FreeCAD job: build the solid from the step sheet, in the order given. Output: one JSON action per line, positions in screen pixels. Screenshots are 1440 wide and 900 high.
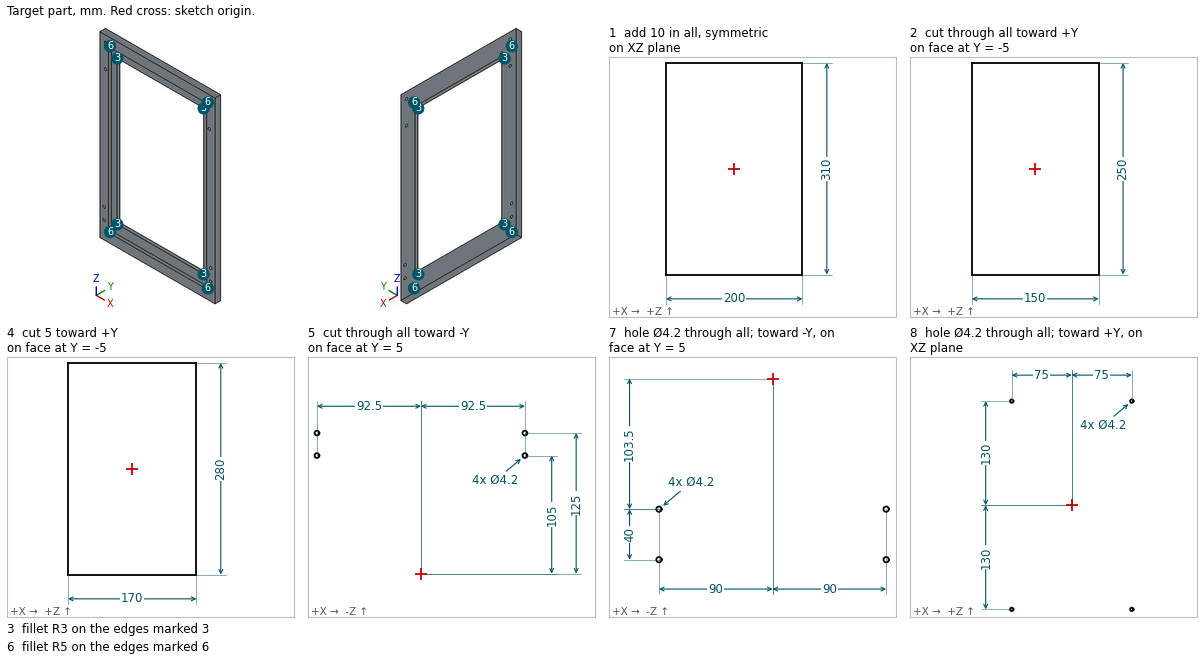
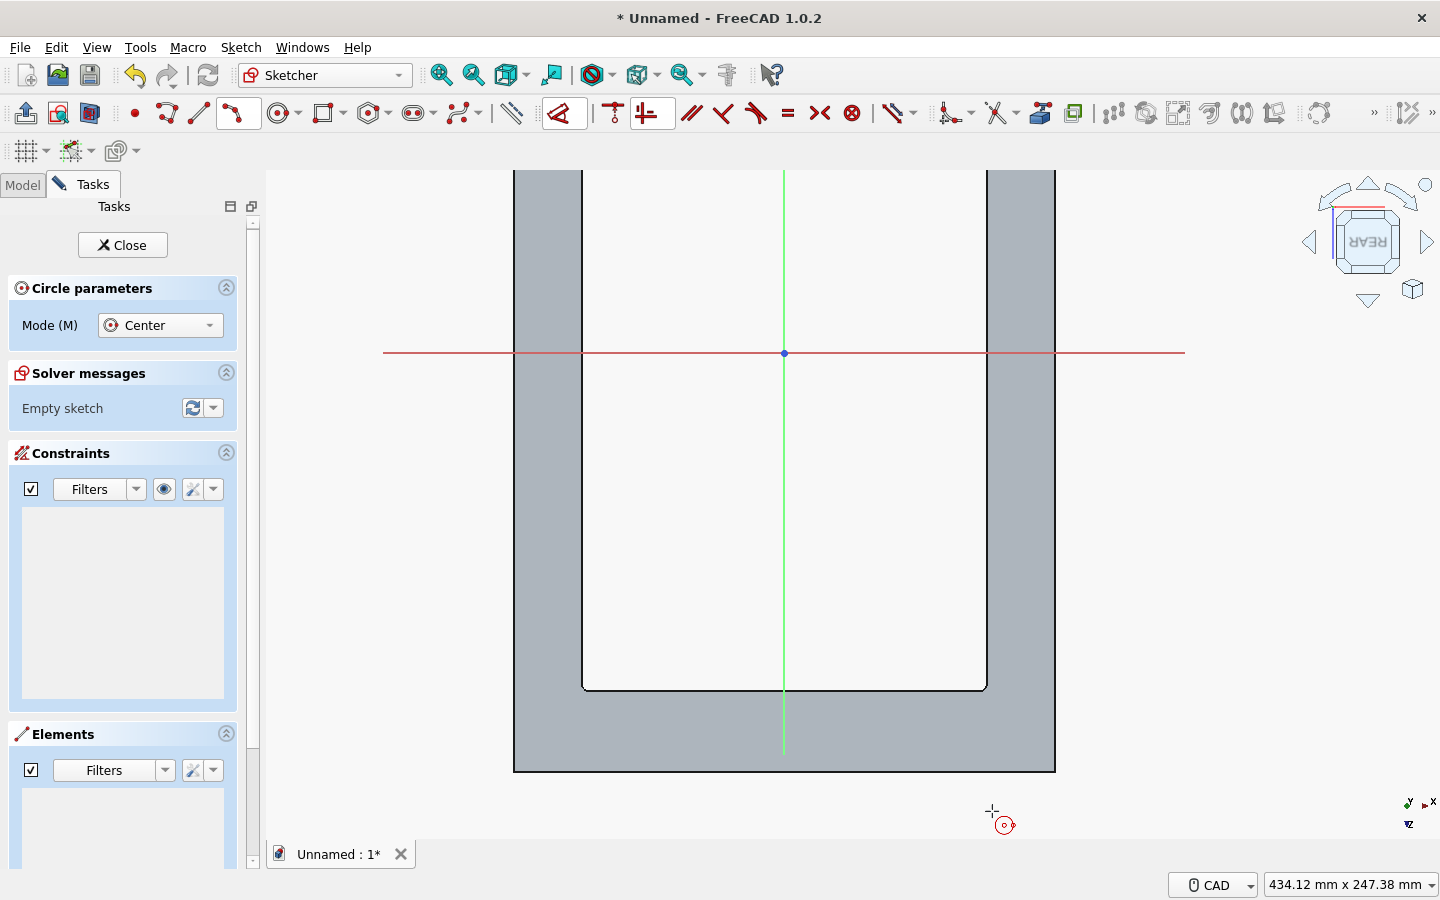
{"action": "scroll", "coordinate": [541, 633], "scroll_direction": "up", "scroll_amount": 7}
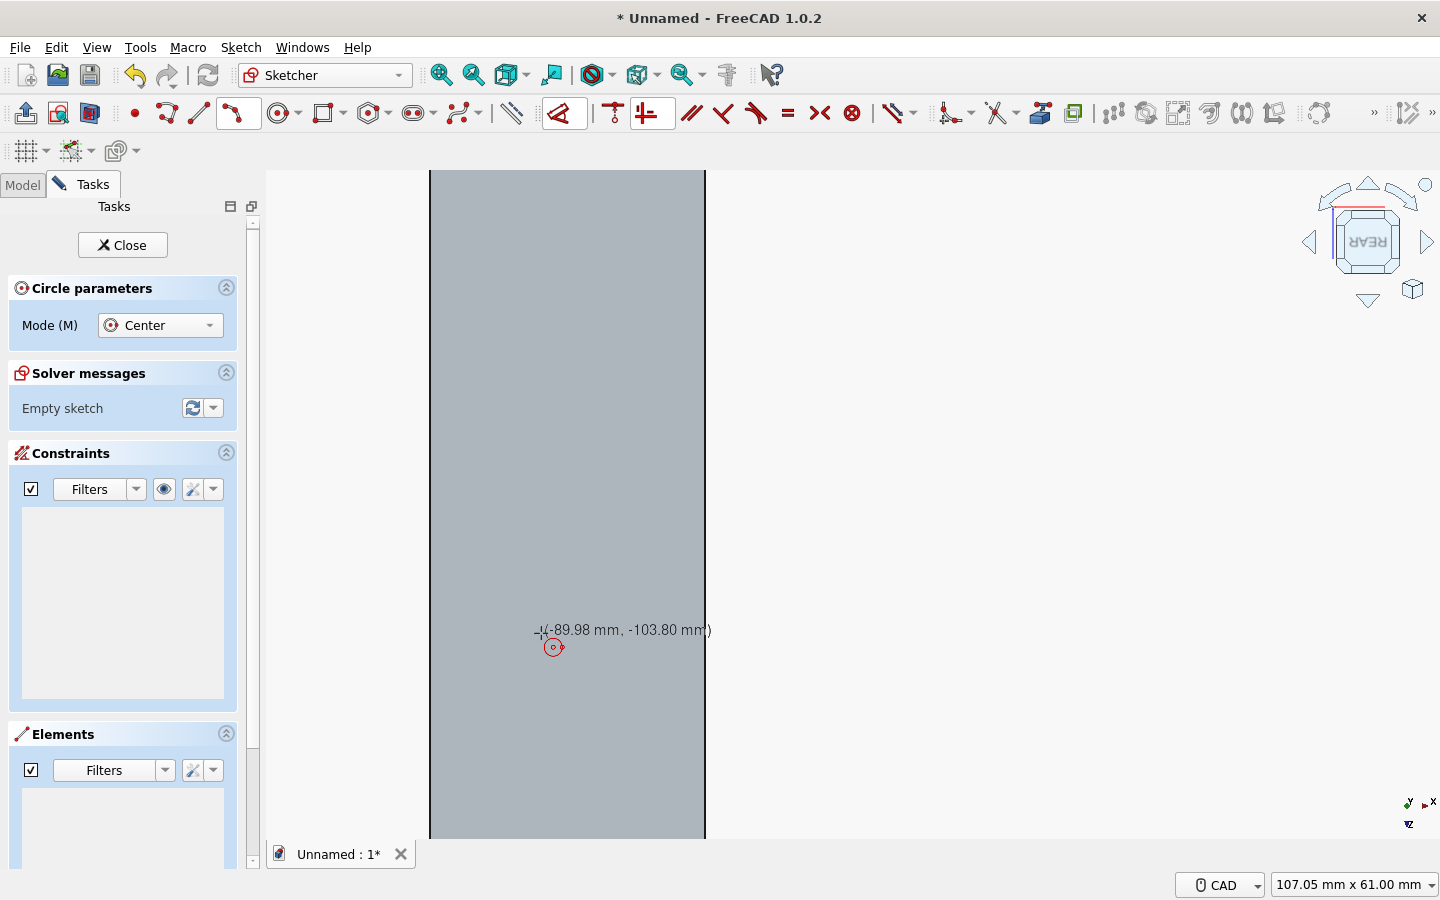
{"action": "scroll", "coordinate": [541, 573], "scroll_direction": "down", "scroll_amount": 7}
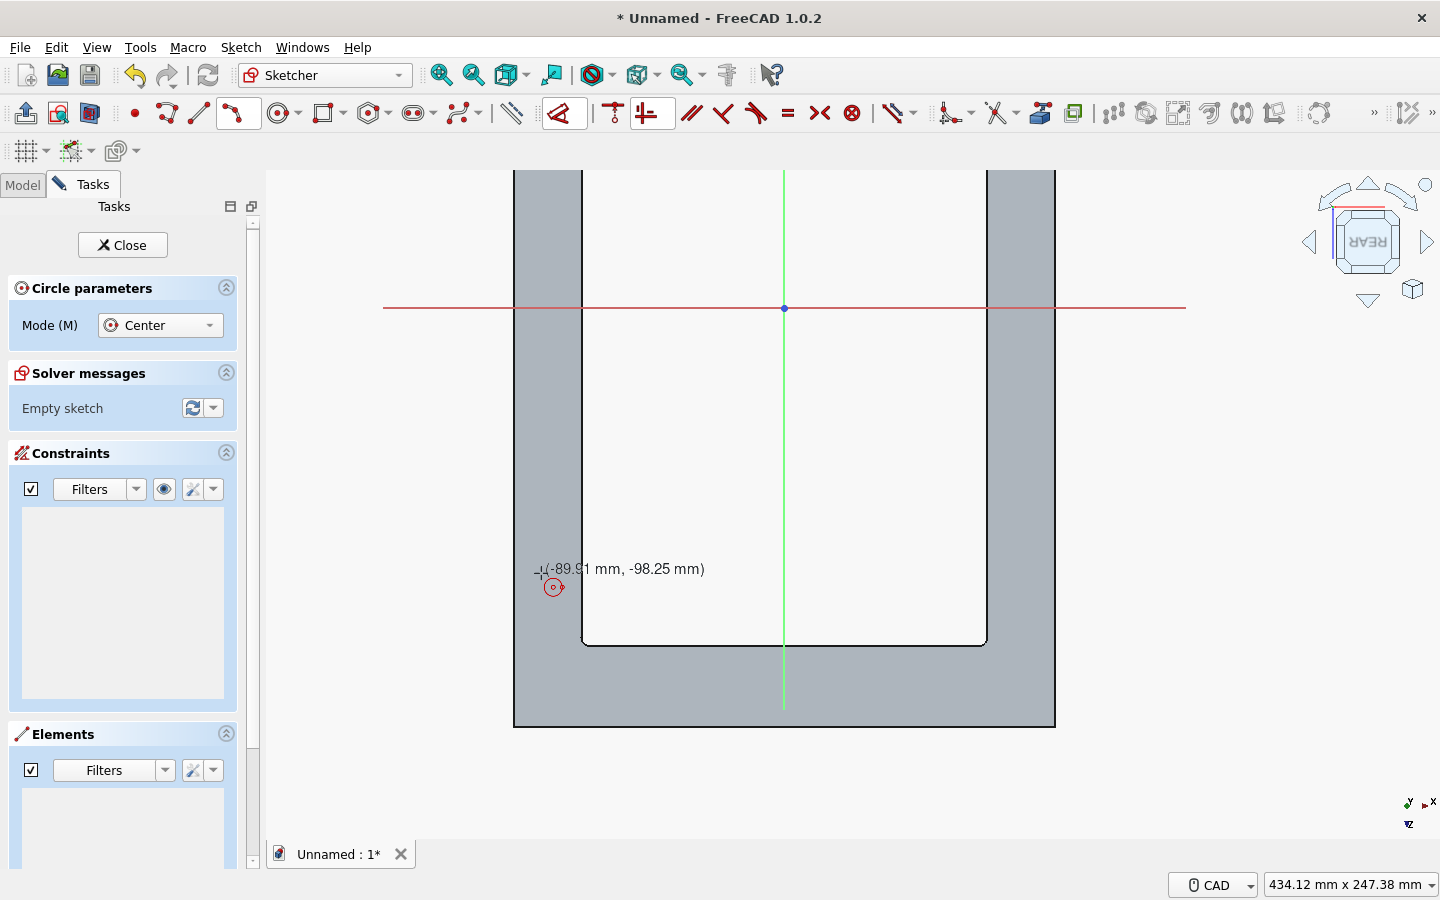
{"action": "left_click", "coordinate": [541, 588]}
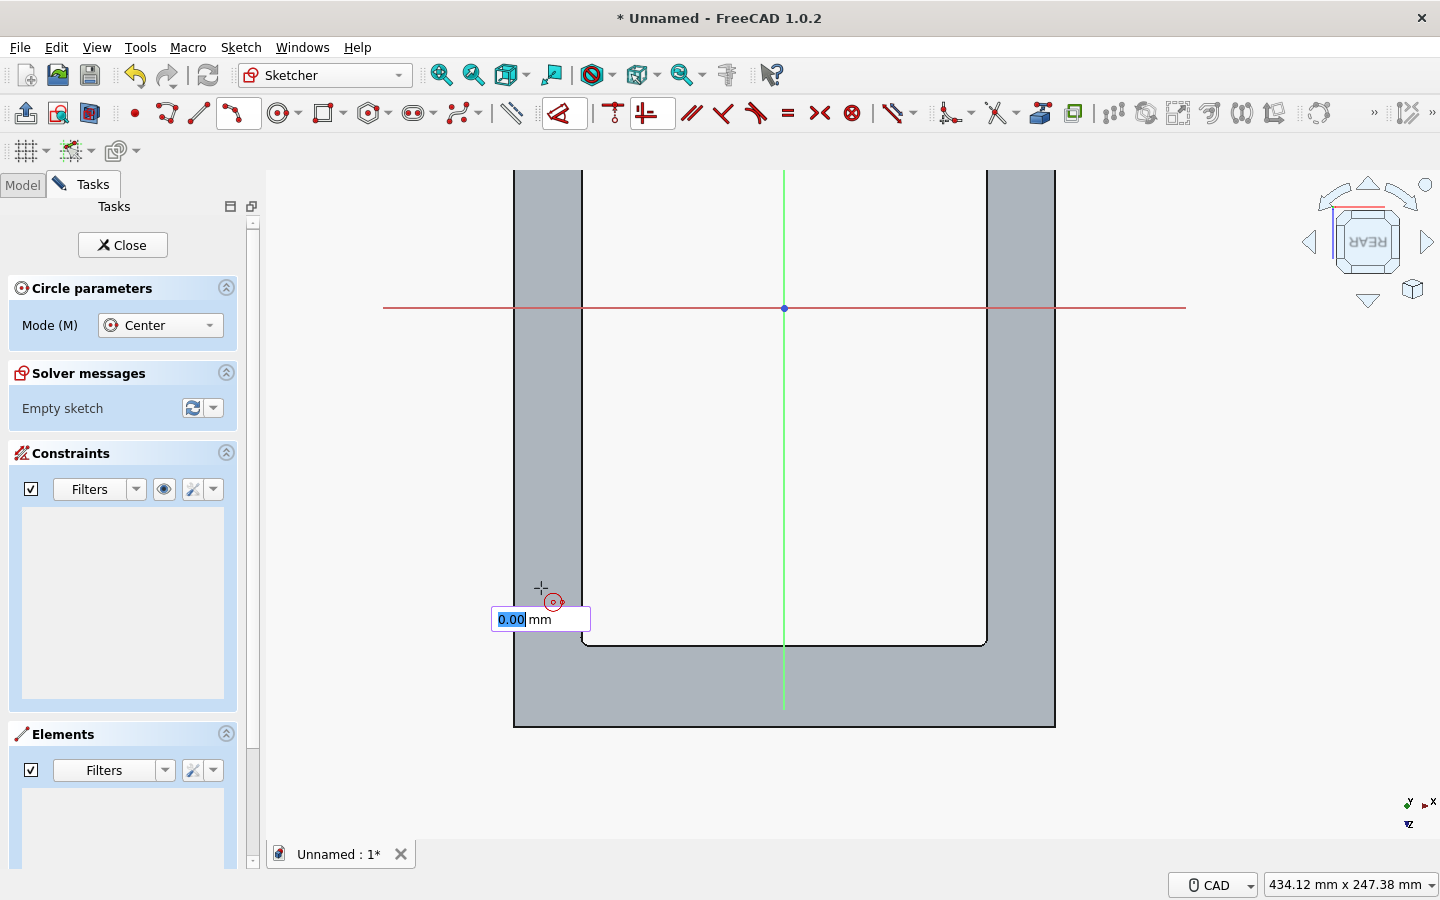
{"action": "scroll", "coordinate": [545, 584], "scroll_direction": "up", "scroll_amount": 6}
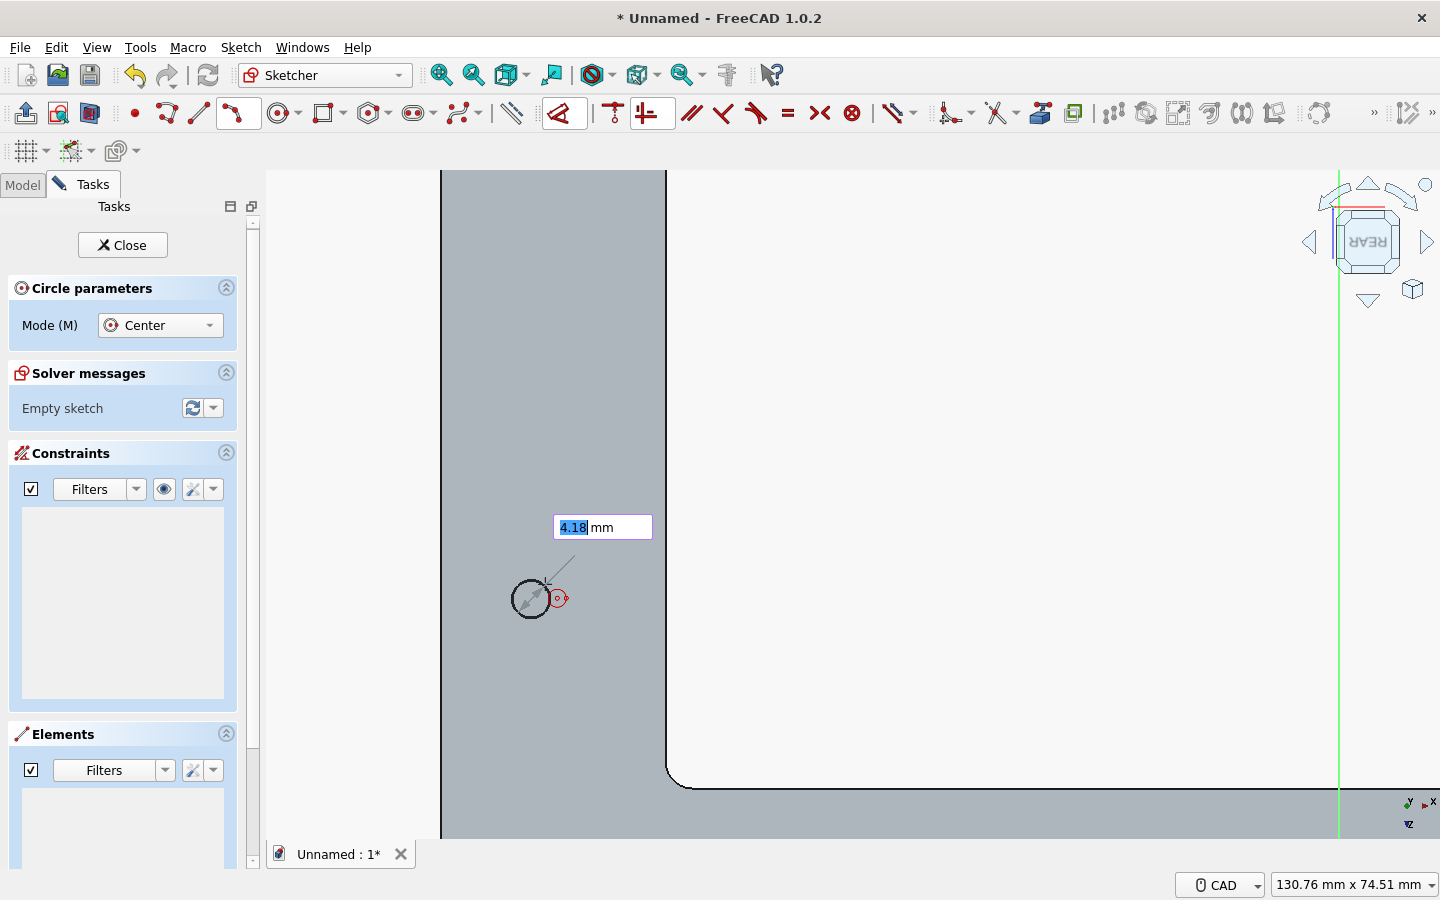
{"action": "left_click", "coordinate": [544, 582]}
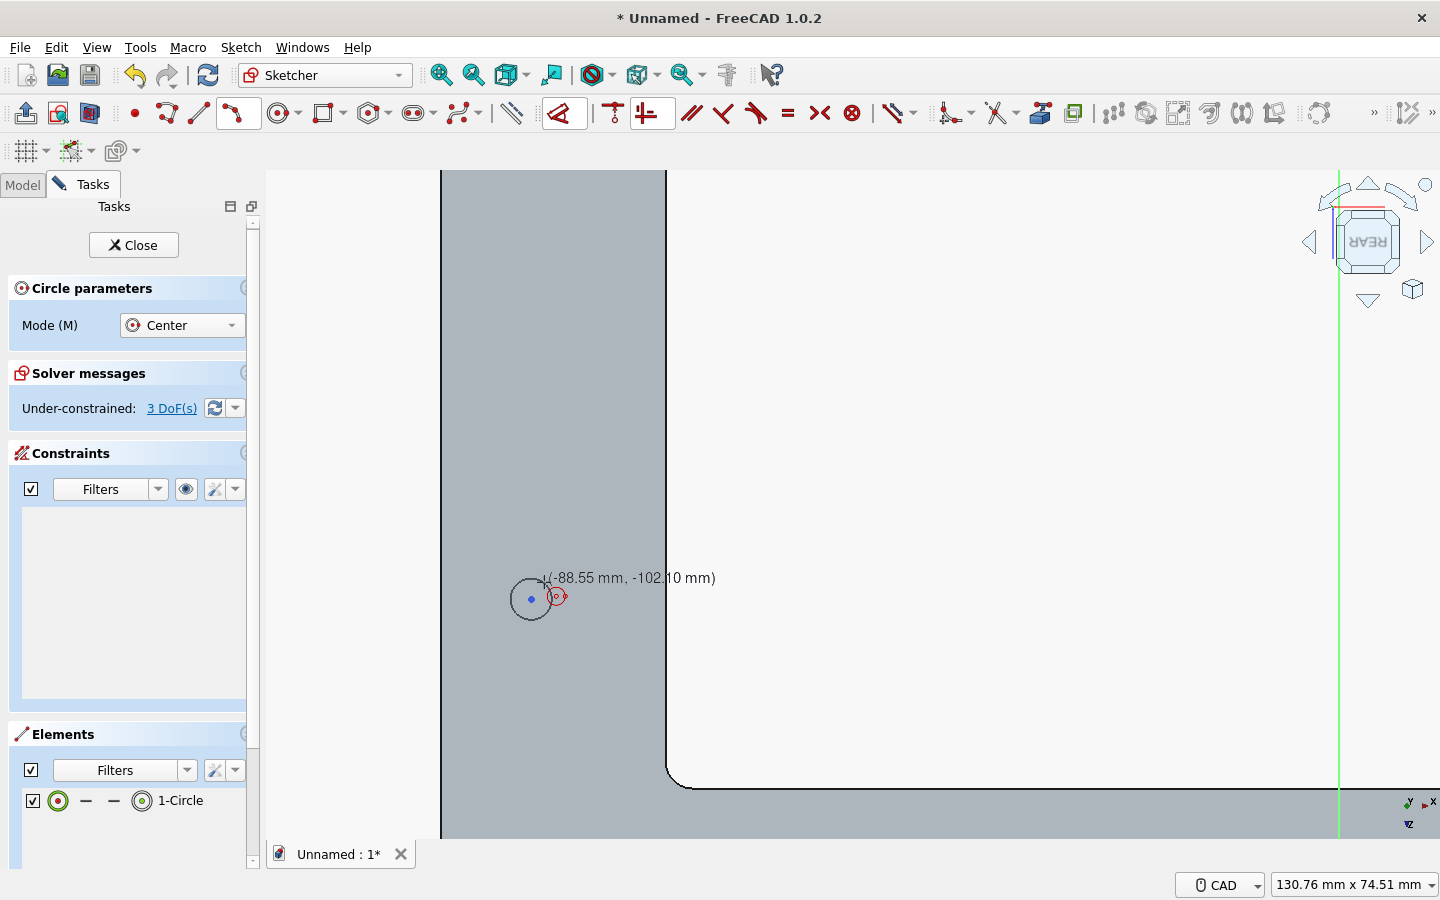
{"action": "scroll", "coordinate": [545, 584], "scroll_direction": "down", "scroll_amount": 6}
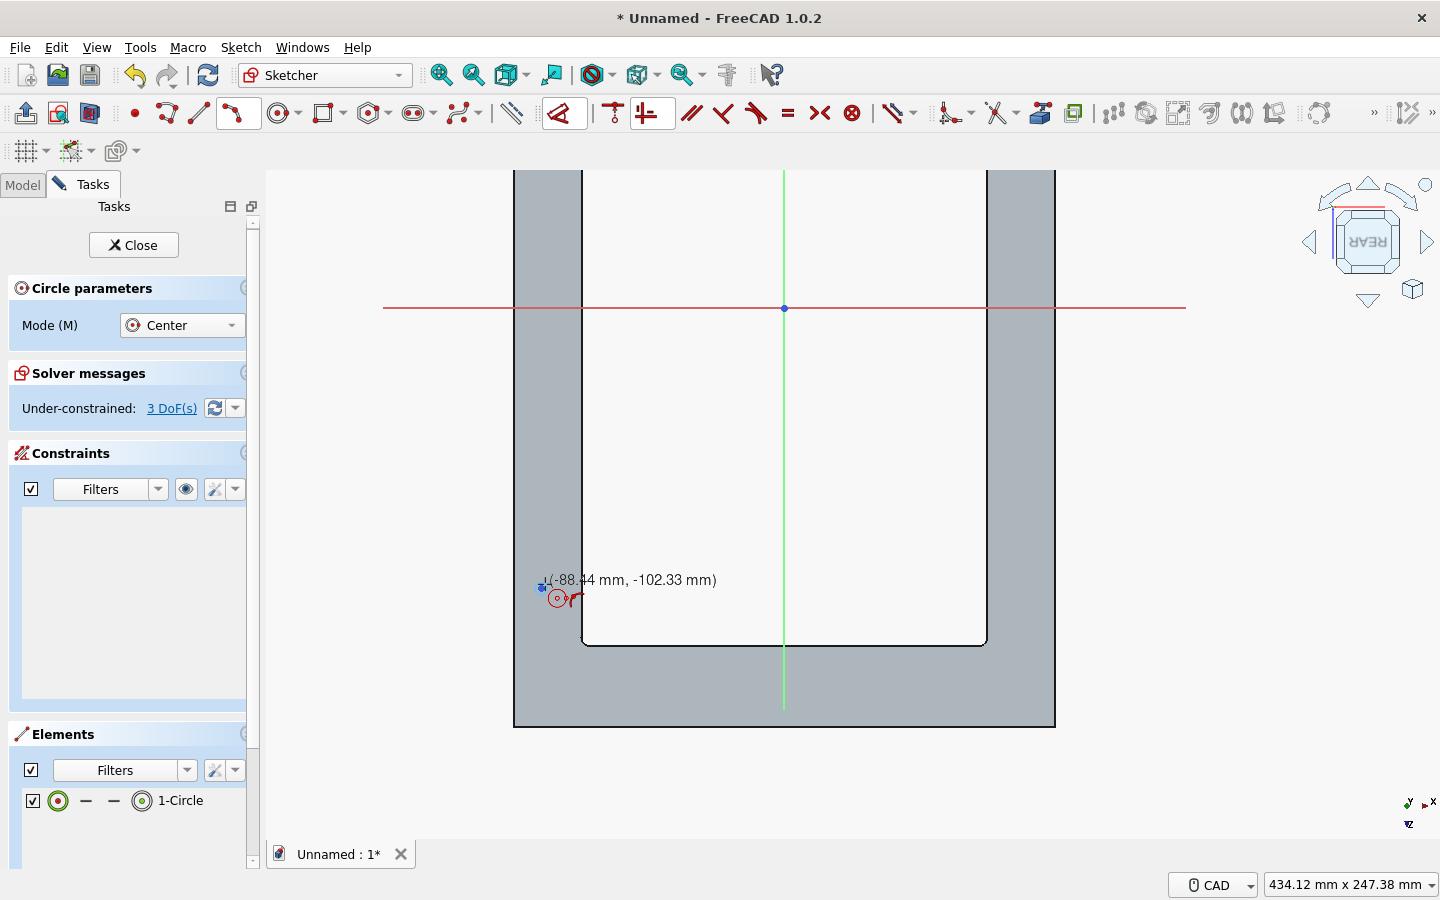
{"action": "scroll", "coordinate": [541, 696], "scroll_direction": "up", "scroll_amount": 7}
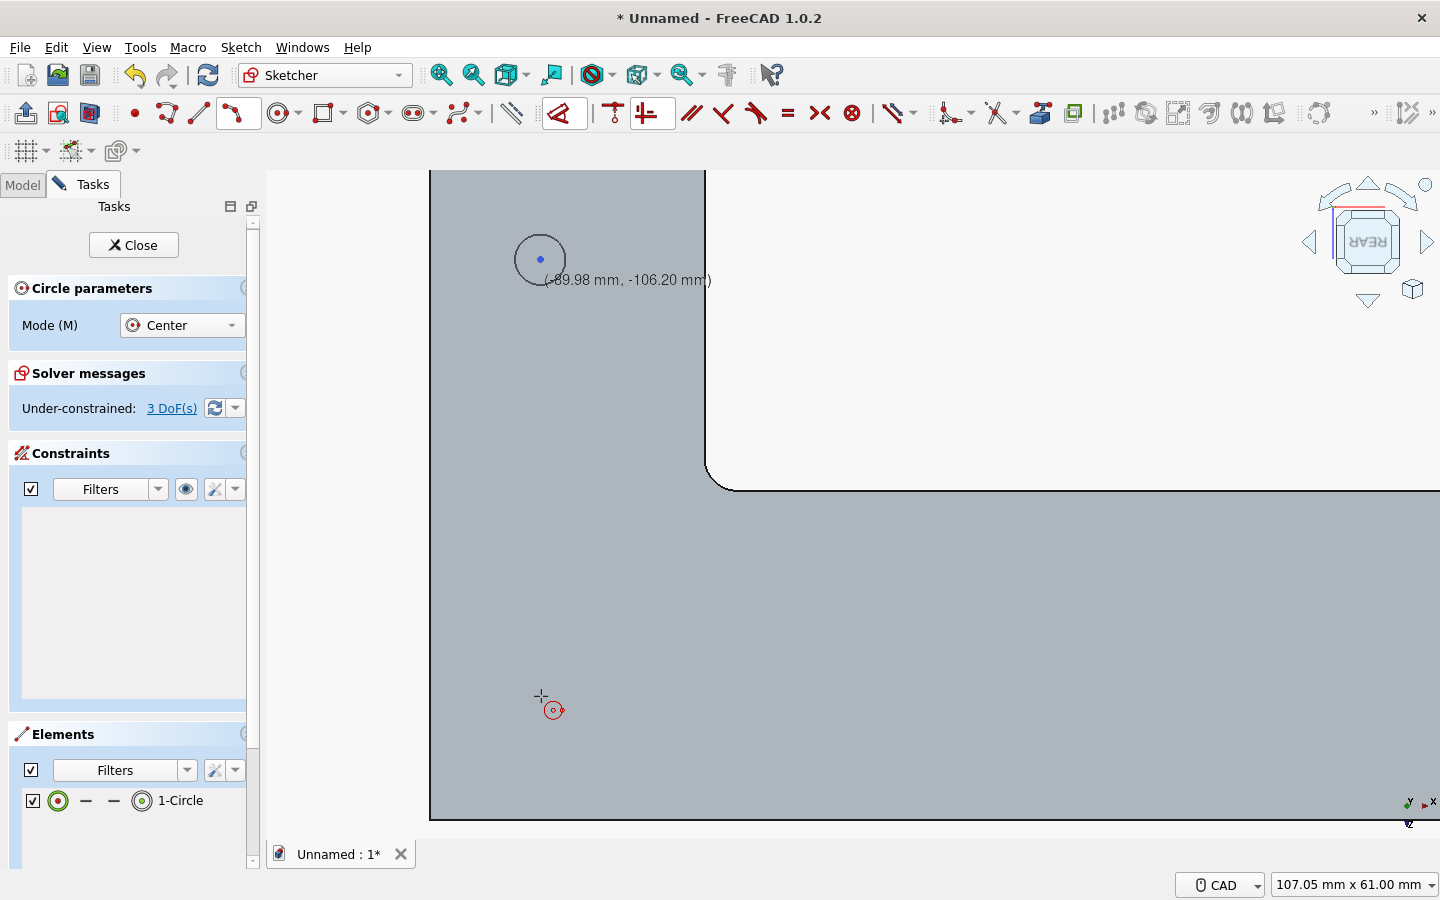
{"action": "scroll", "coordinate": [541, 696], "scroll_direction": "down", "scroll_amount": 7}